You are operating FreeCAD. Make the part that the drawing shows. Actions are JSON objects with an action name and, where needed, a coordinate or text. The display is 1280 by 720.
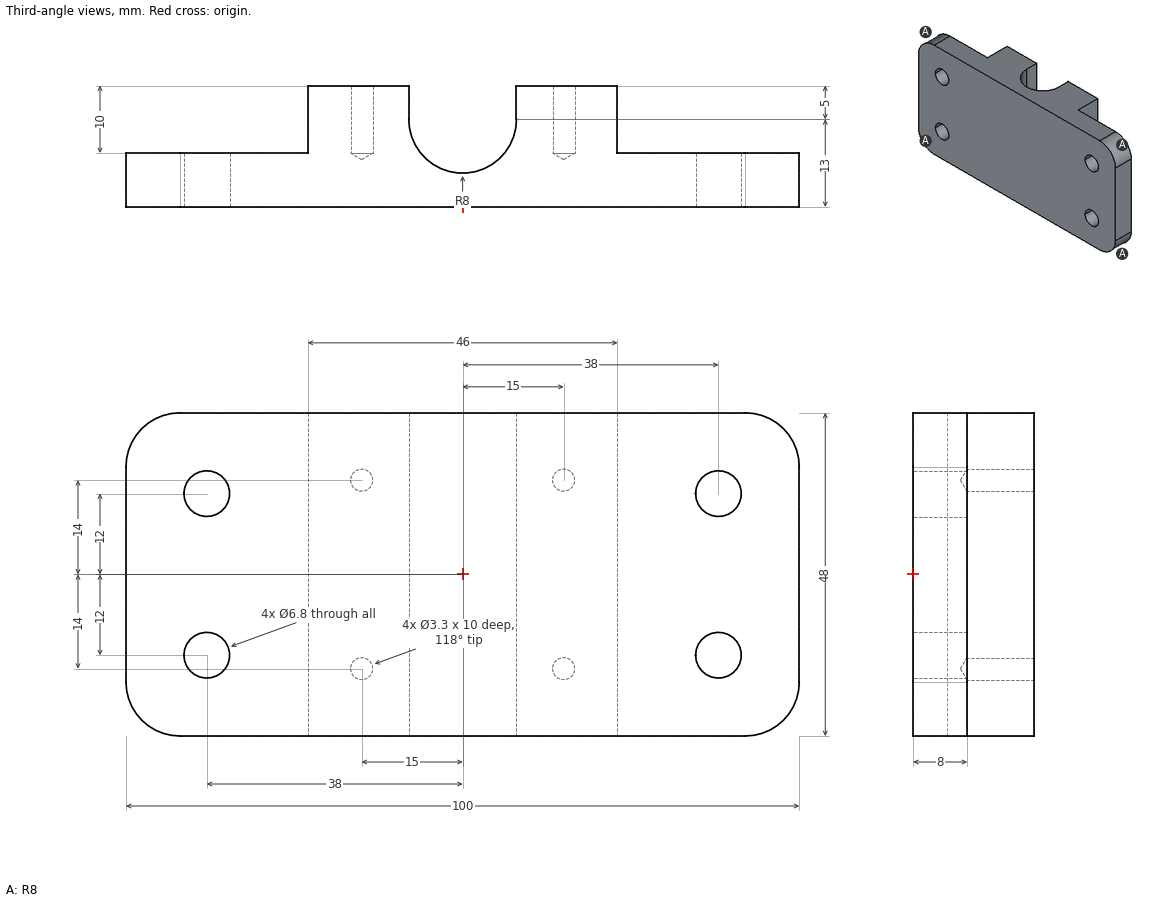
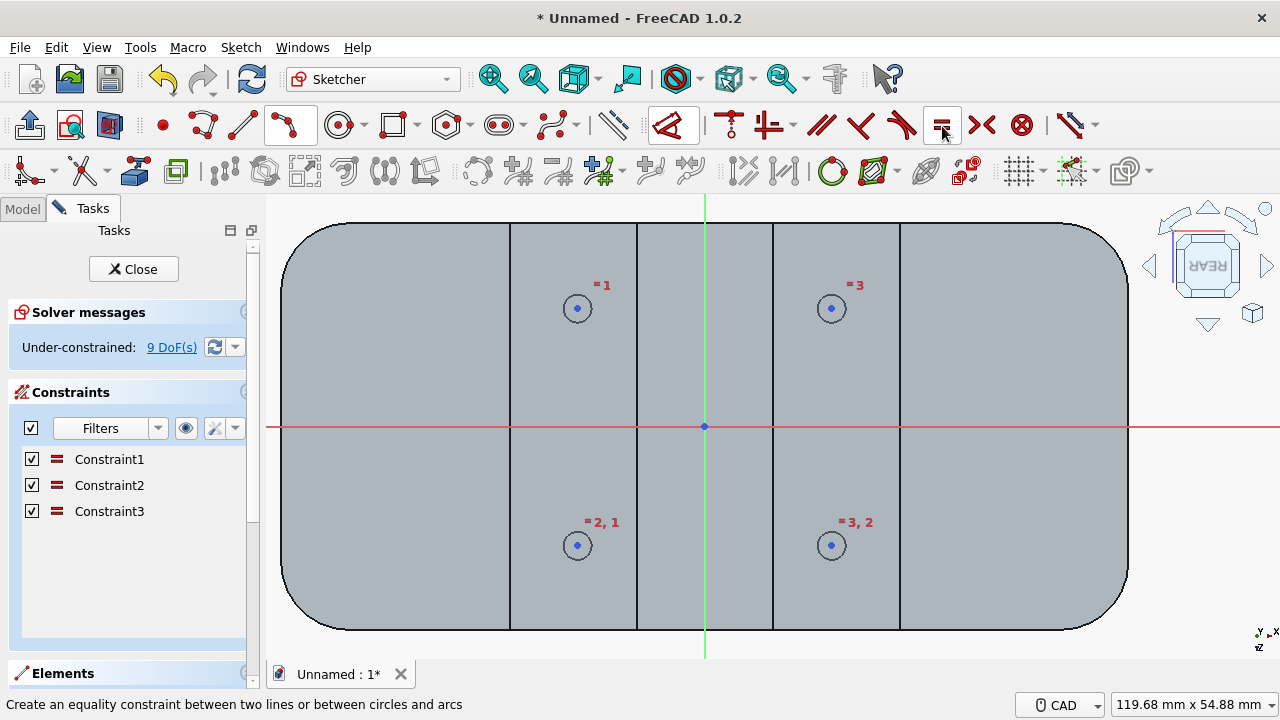
{"action": "left_click", "coordinate": [578, 309]}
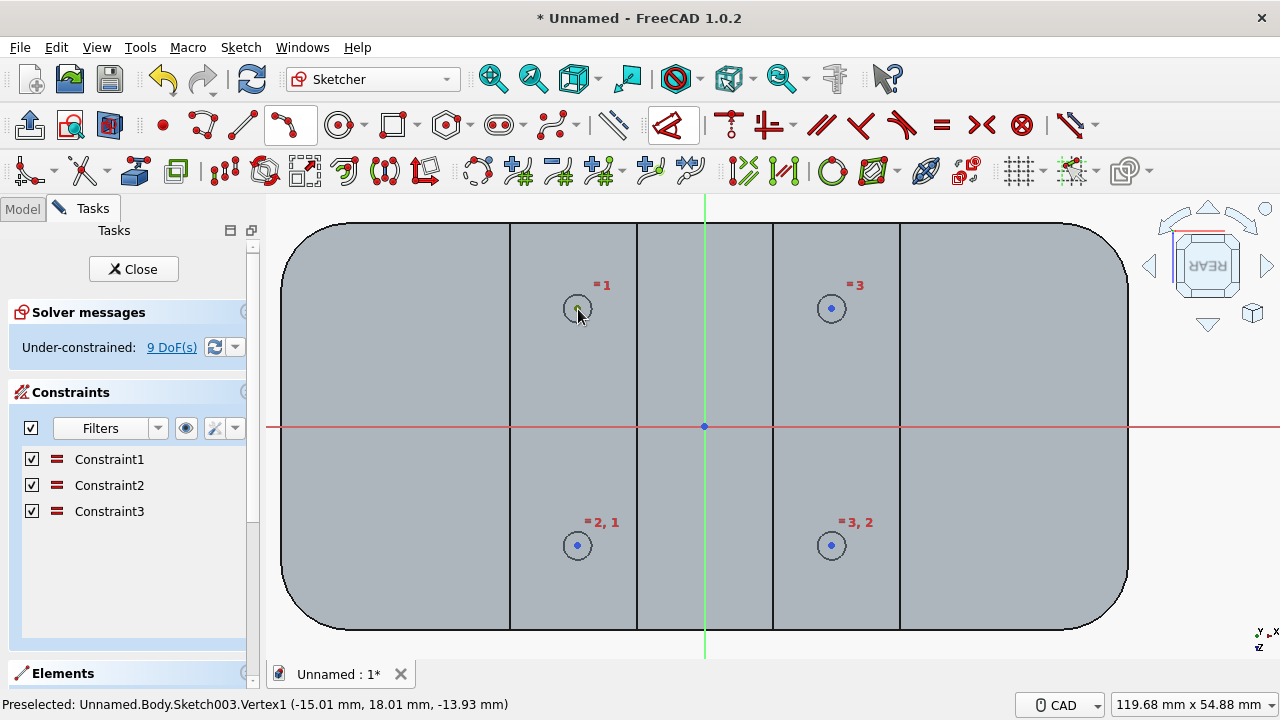
{"action": "left_click", "coordinate": [578, 546]}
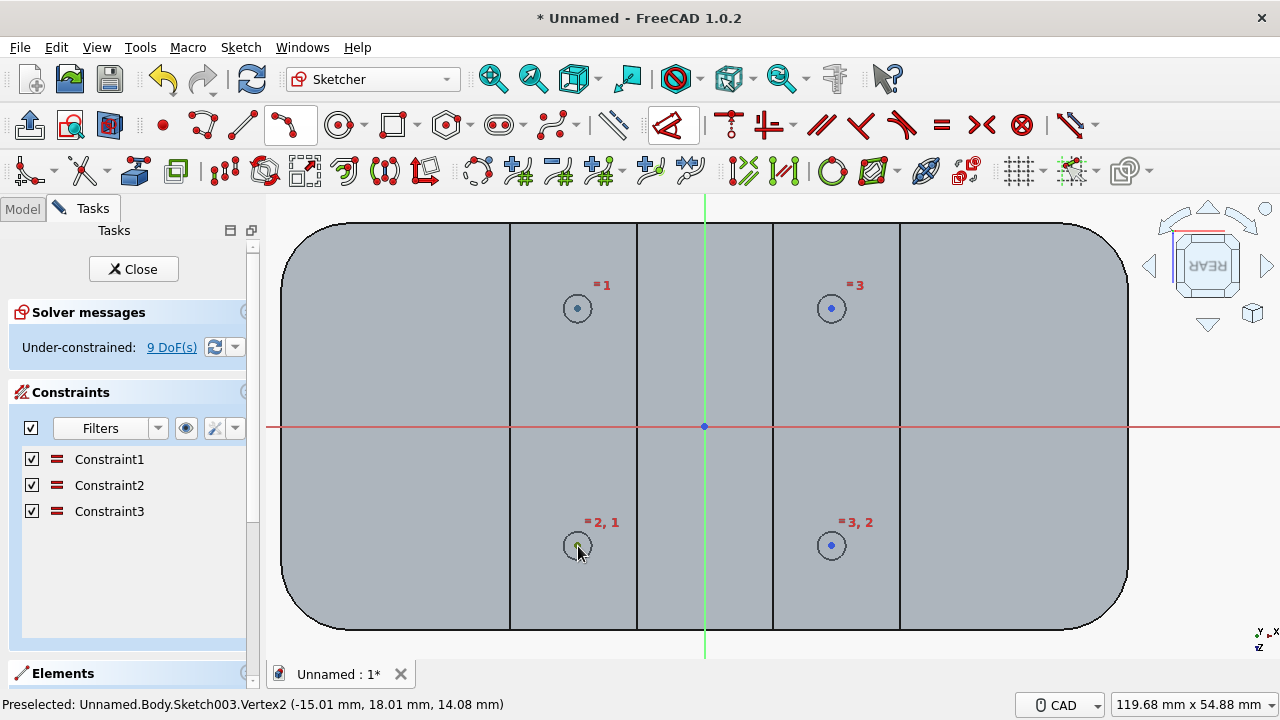
{"action": "key", "text": "v"}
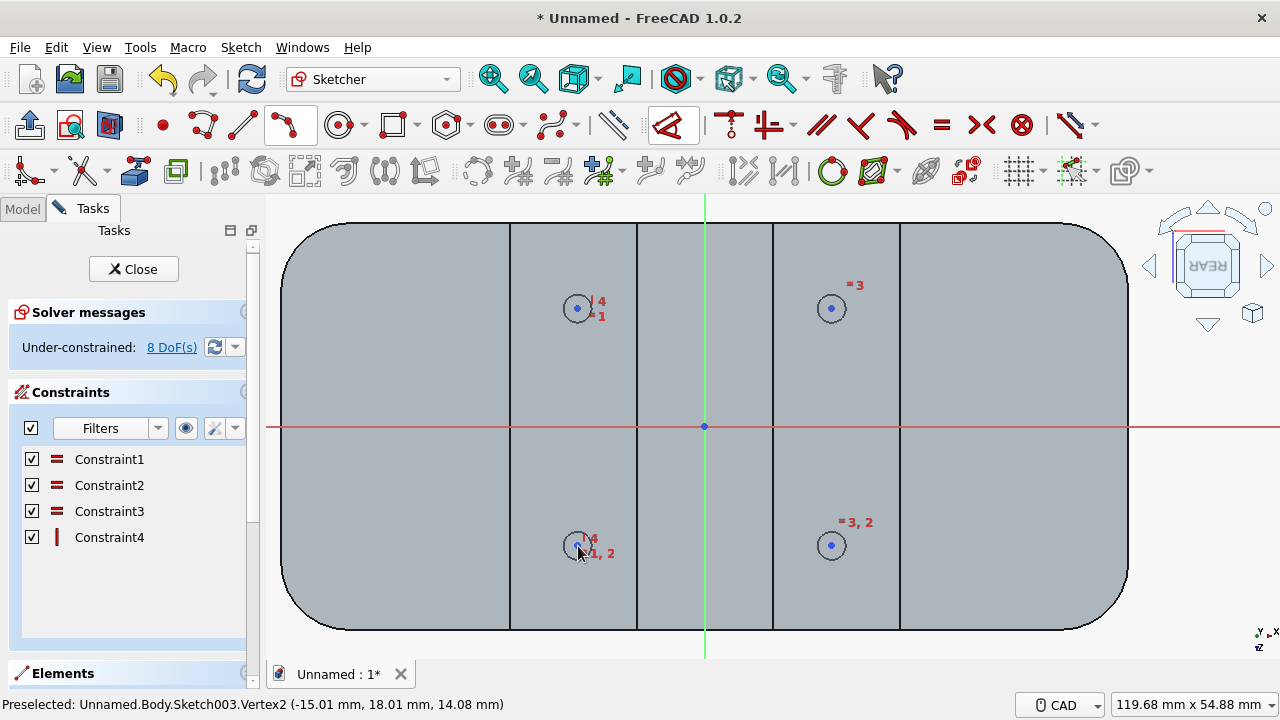
{"action": "left_click", "coordinate": [578, 546]}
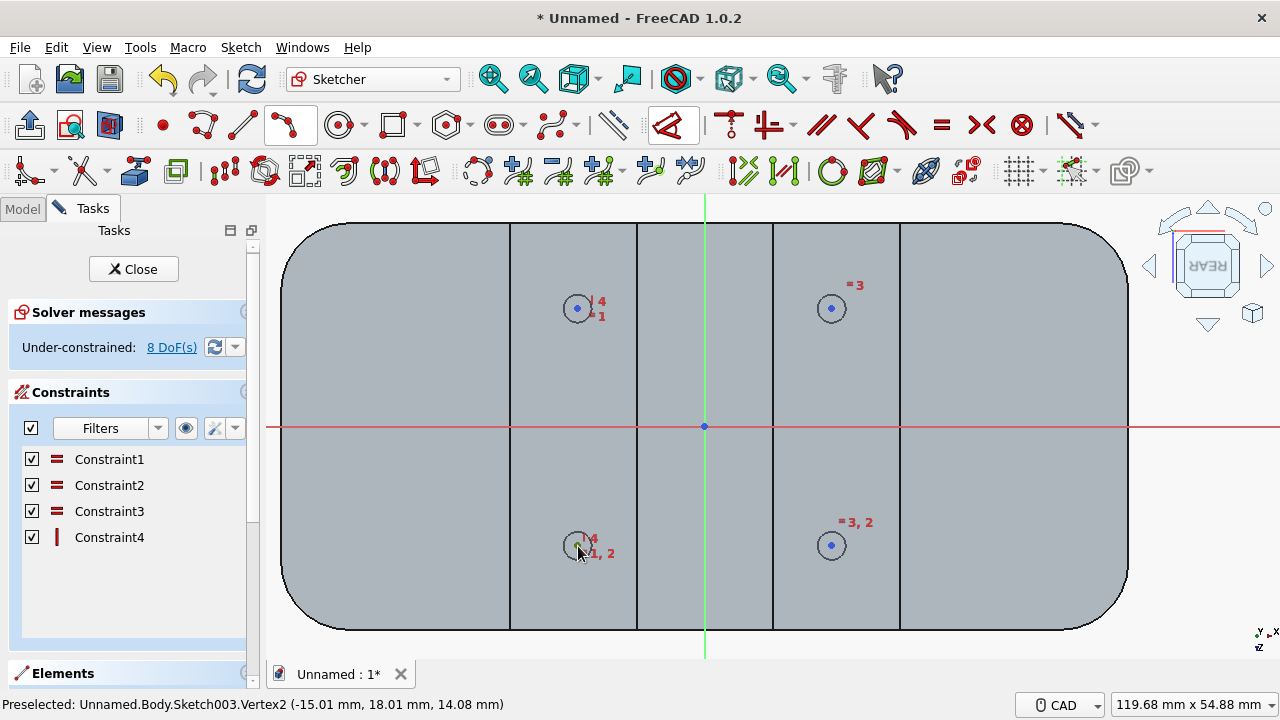
{"action": "left_click", "coordinate": [832, 546]}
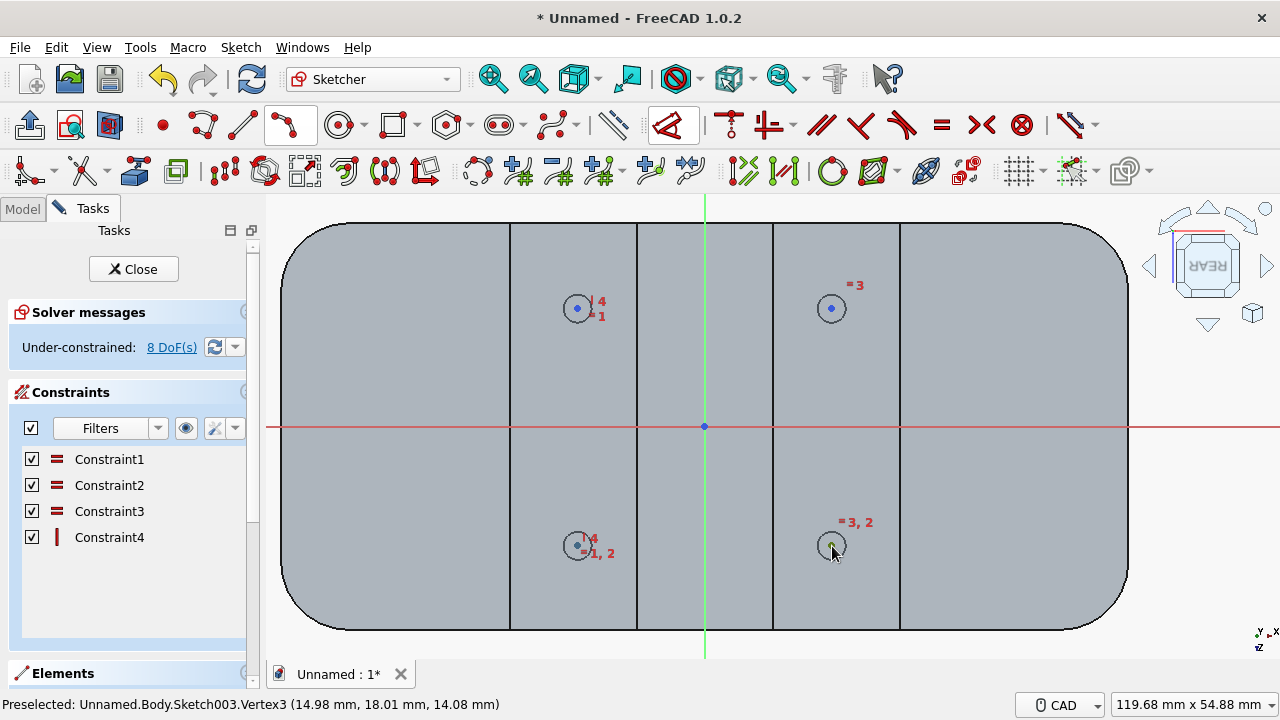
{"action": "left_click", "coordinate": [796, 126]}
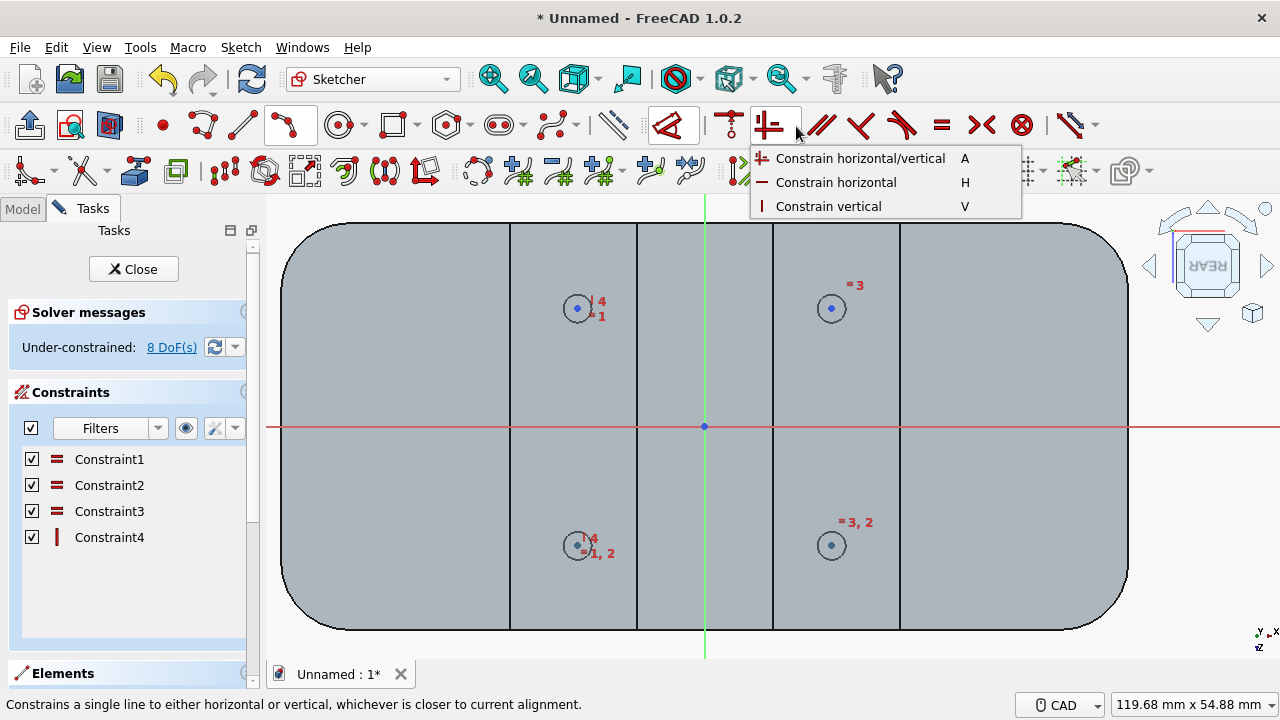
{"action": "left_click", "coordinate": [886, 182]}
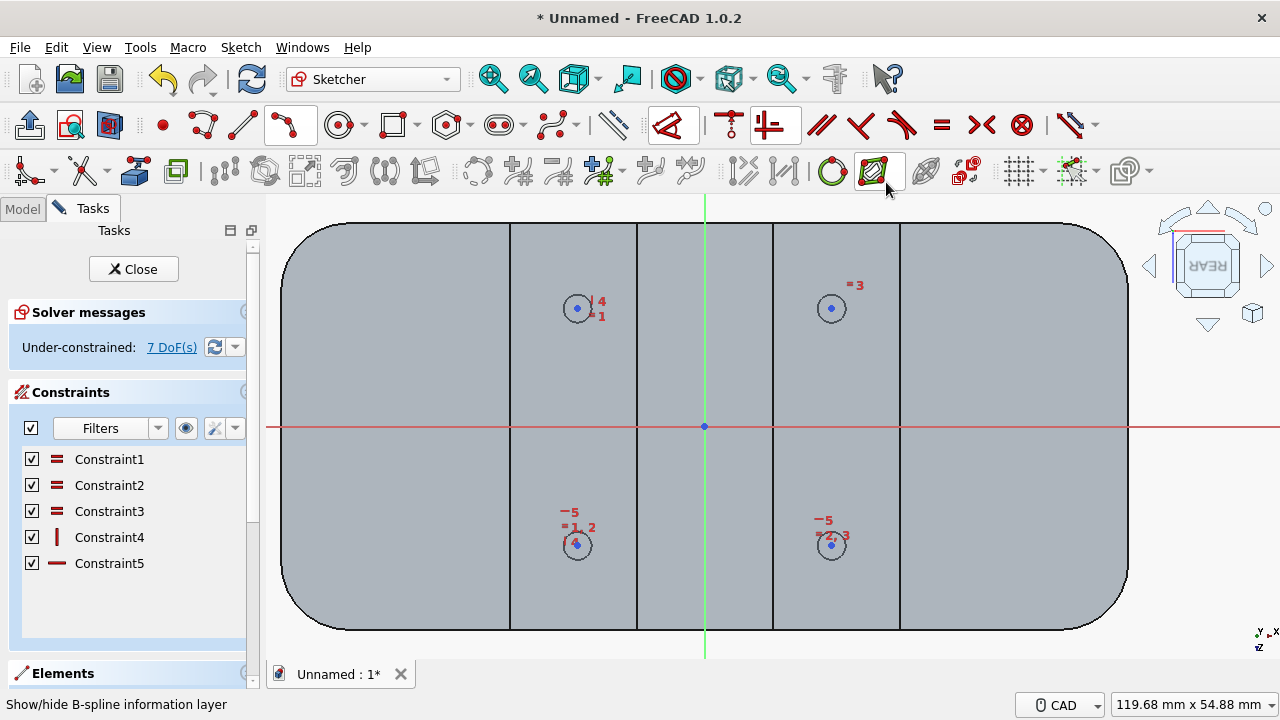
{"action": "left_click", "coordinate": [832, 546]}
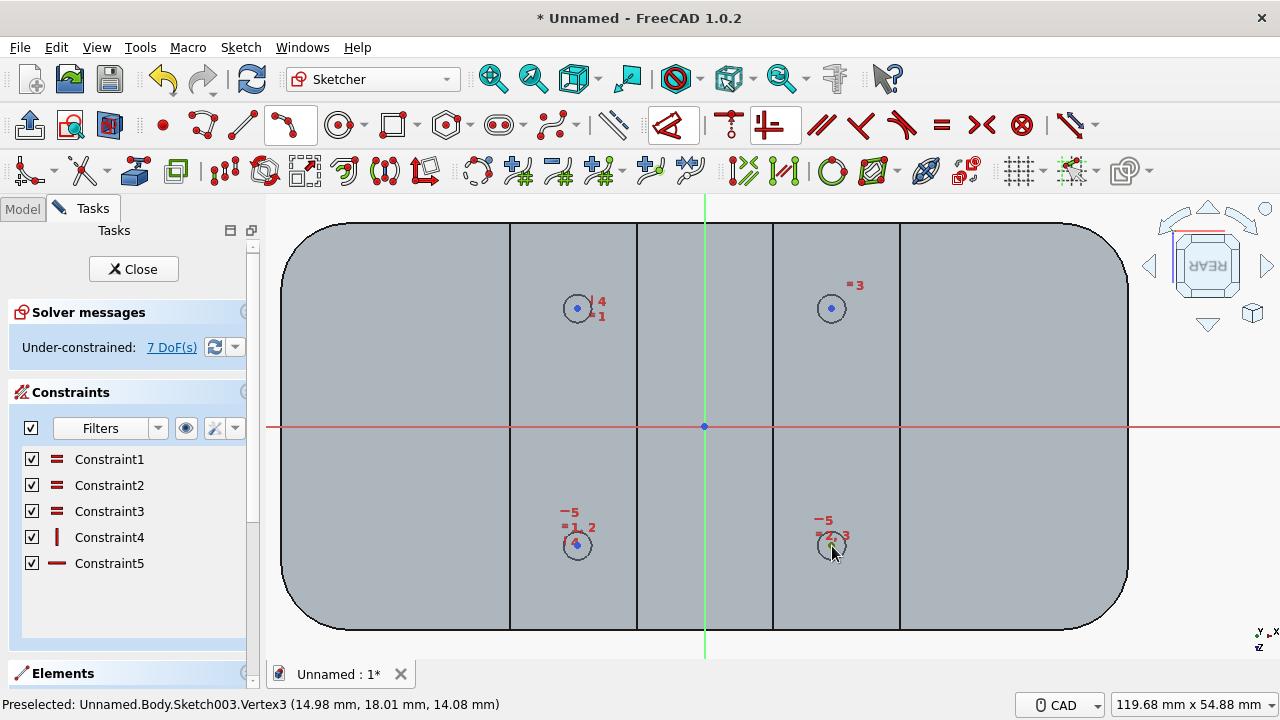
{"action": "left_click", "coordinate": [832, 309]}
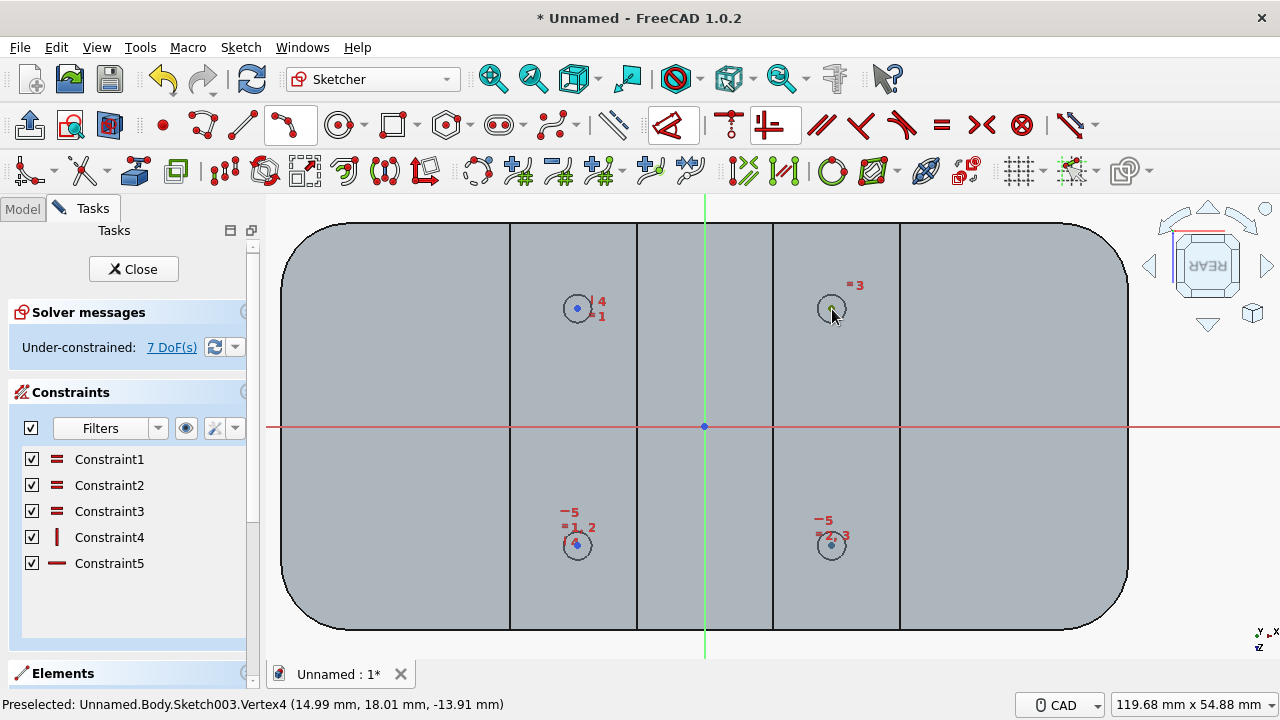
{"action": "key", "text": "v"}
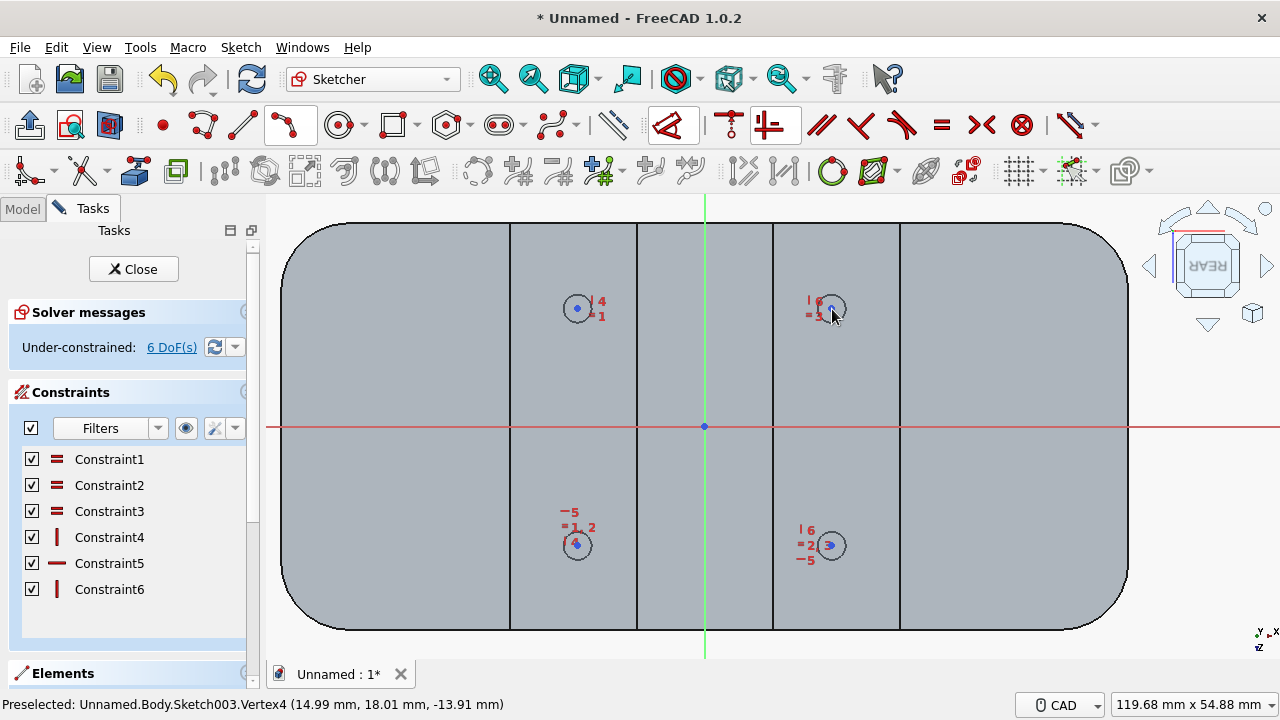
{"action": "left_click", "coordinate": [578, 309]}